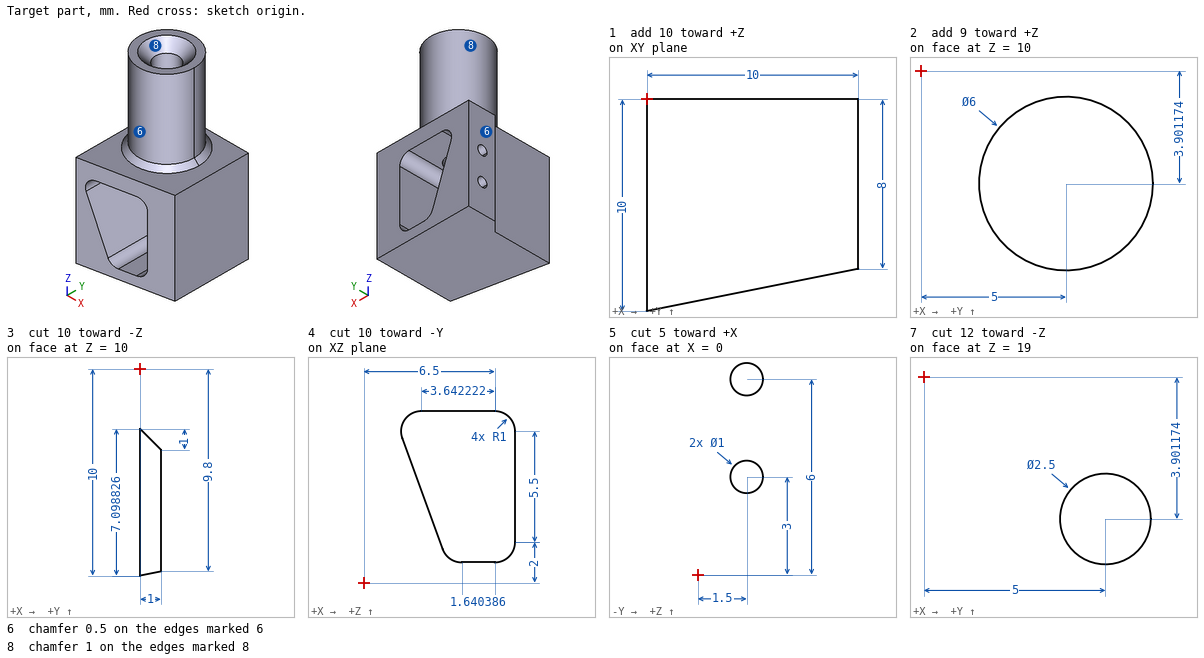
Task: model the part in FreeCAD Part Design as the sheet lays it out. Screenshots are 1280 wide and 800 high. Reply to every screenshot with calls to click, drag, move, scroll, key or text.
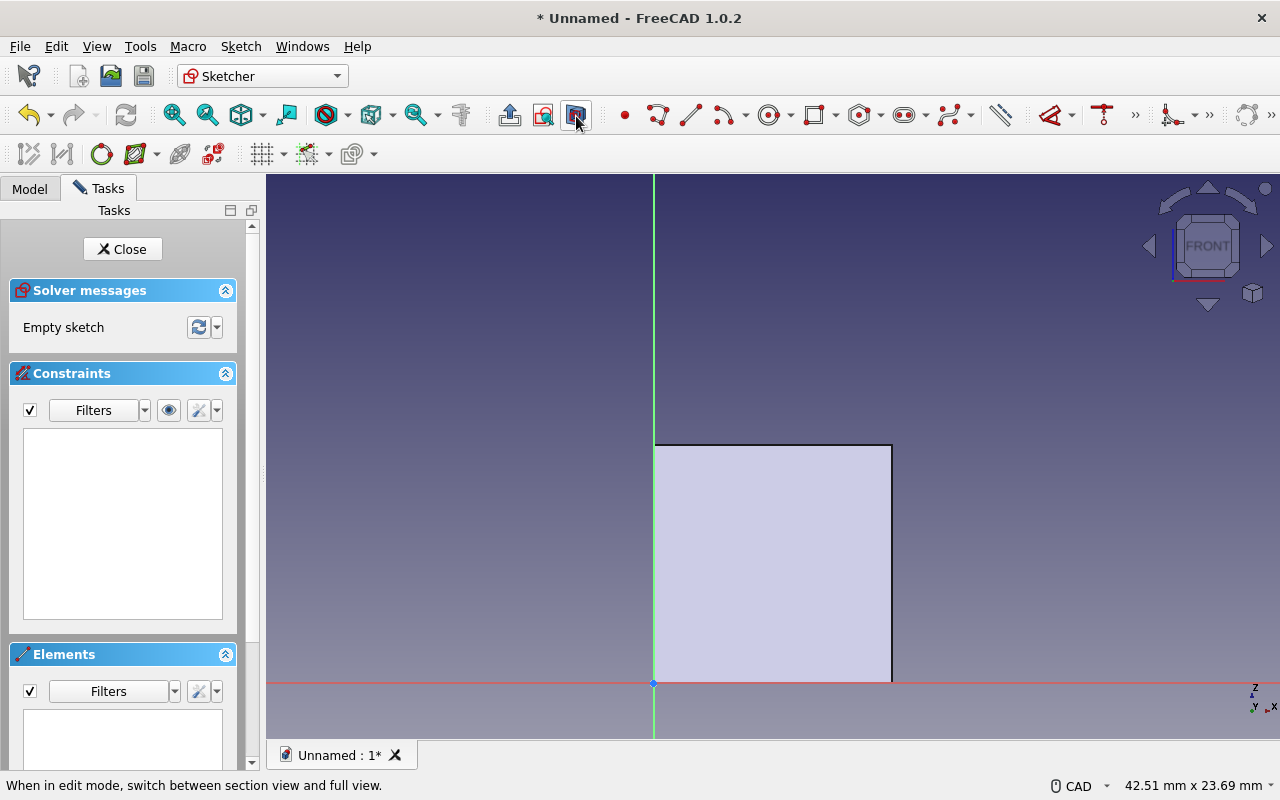
scroll(790, 711, up, 3)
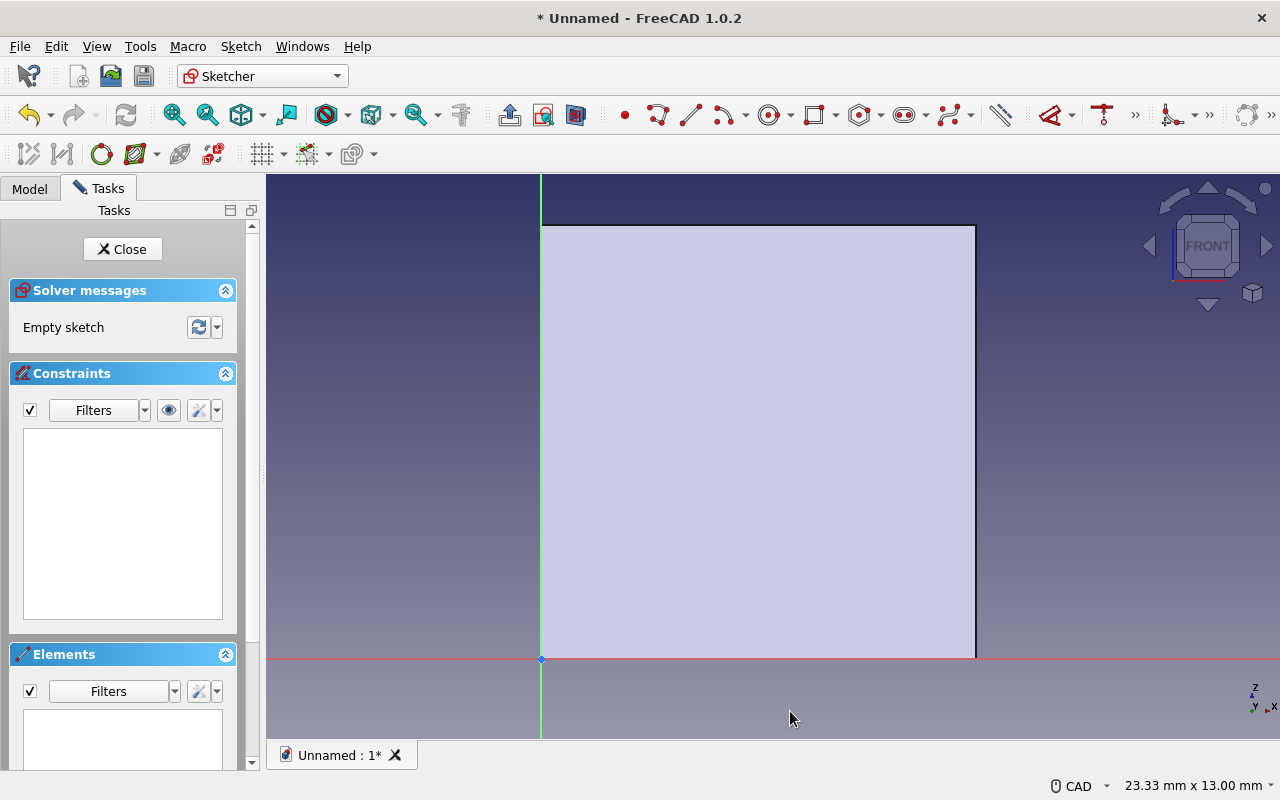
click(691, 116)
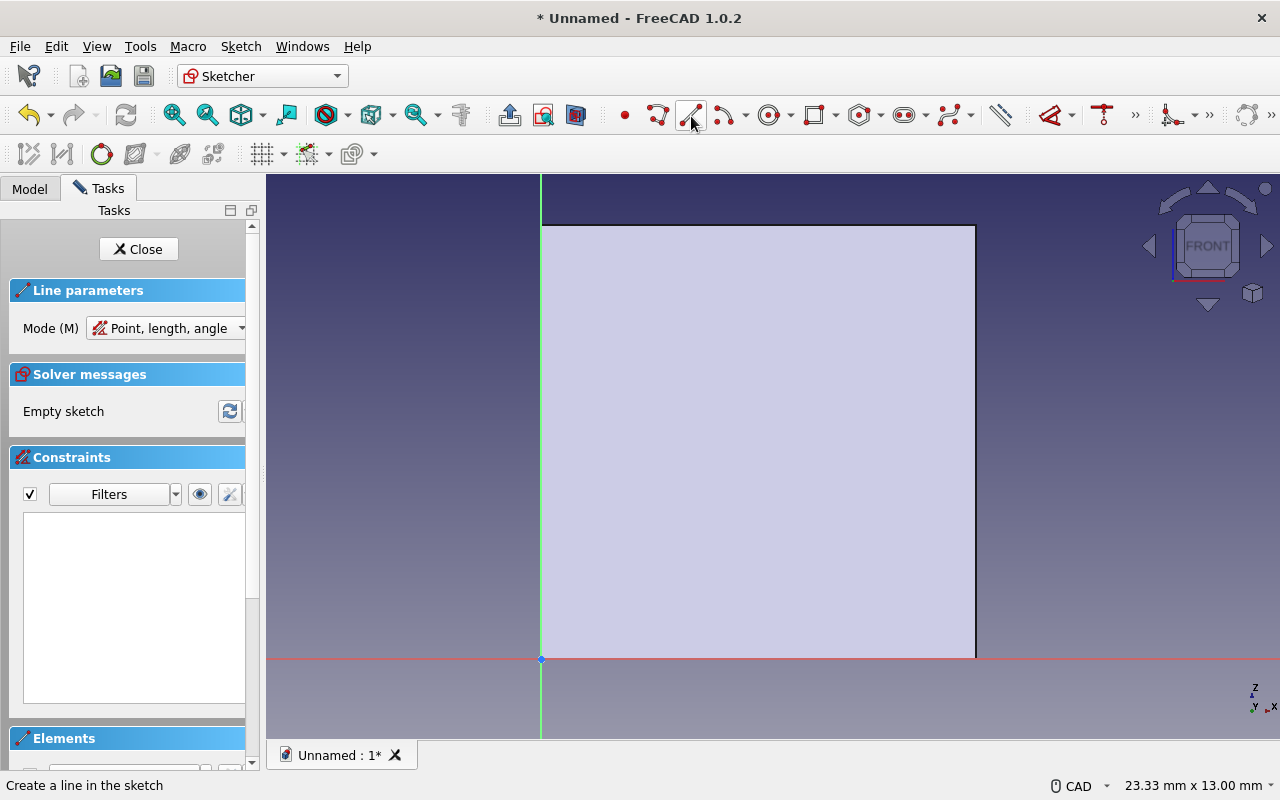
click(712, 587)
click(625, 348)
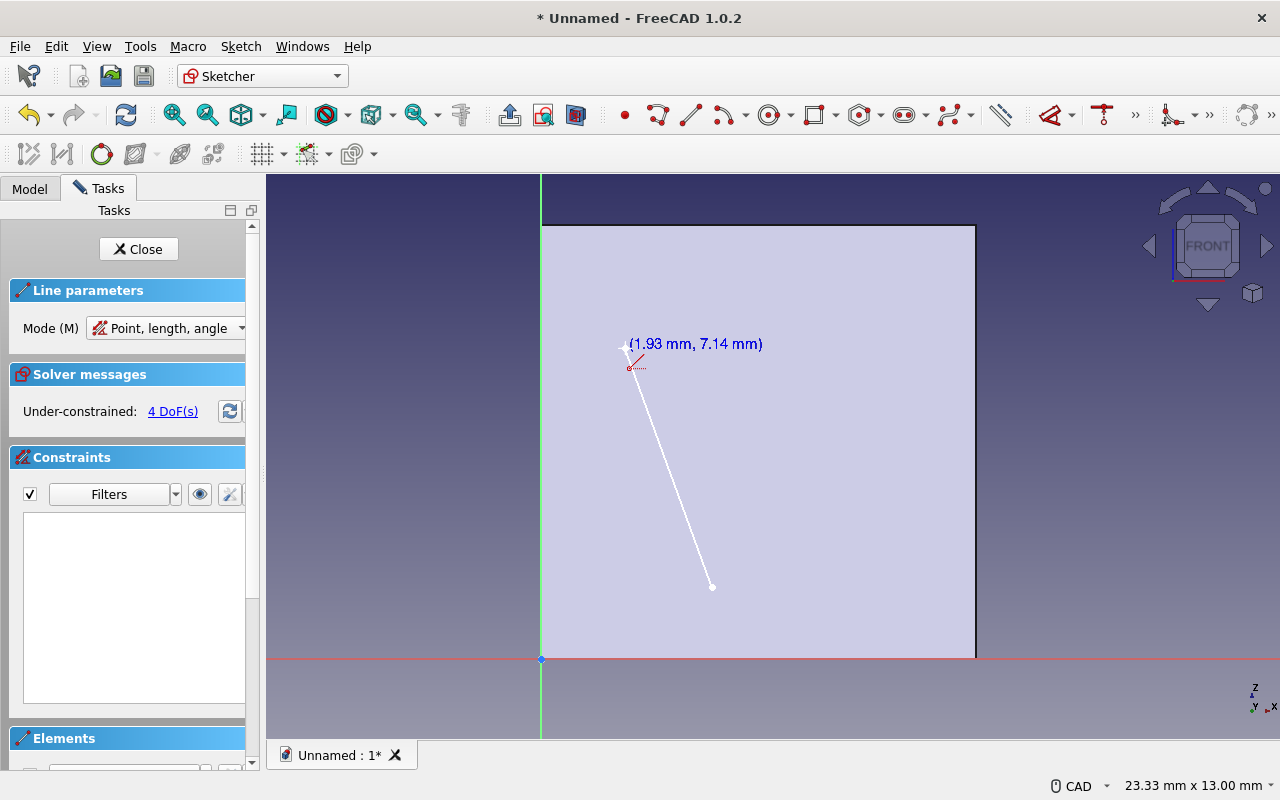
click(665, 290)
click(824, 290)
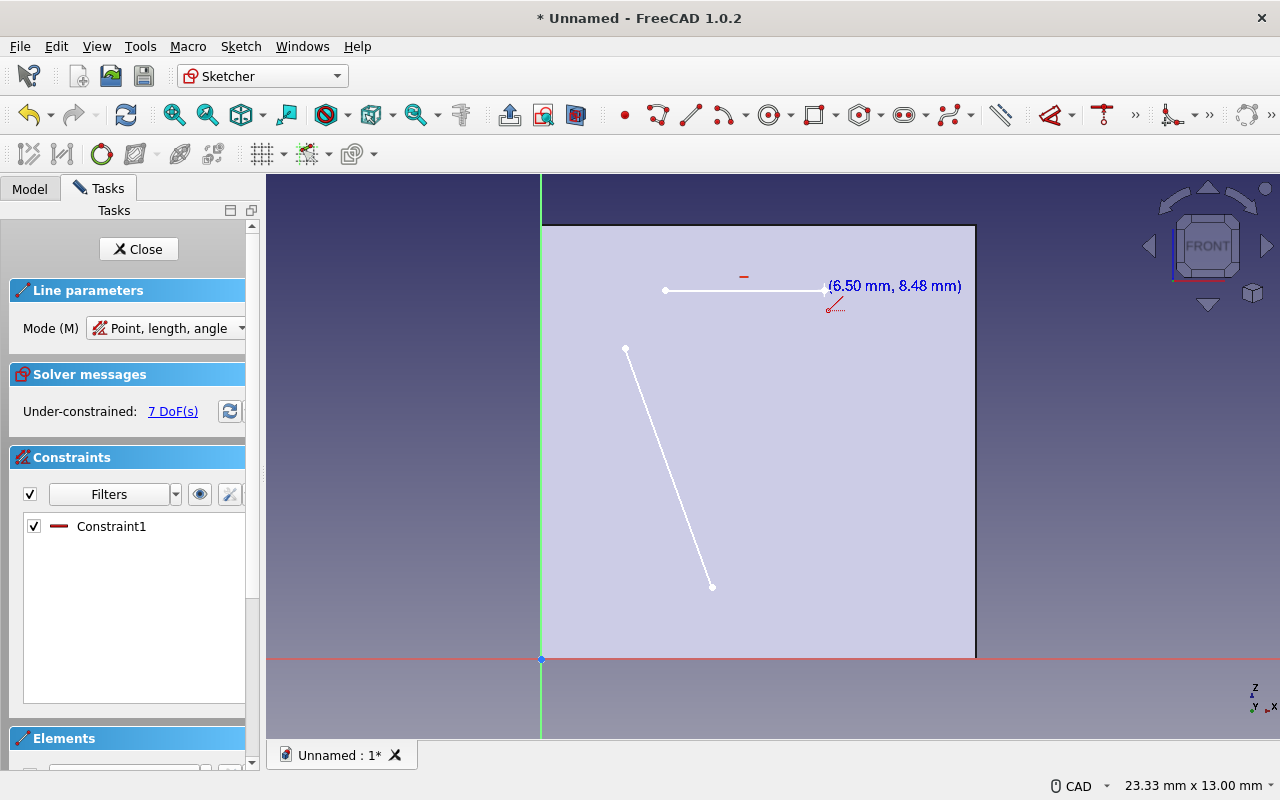
click(867, 333)
click(867, 572)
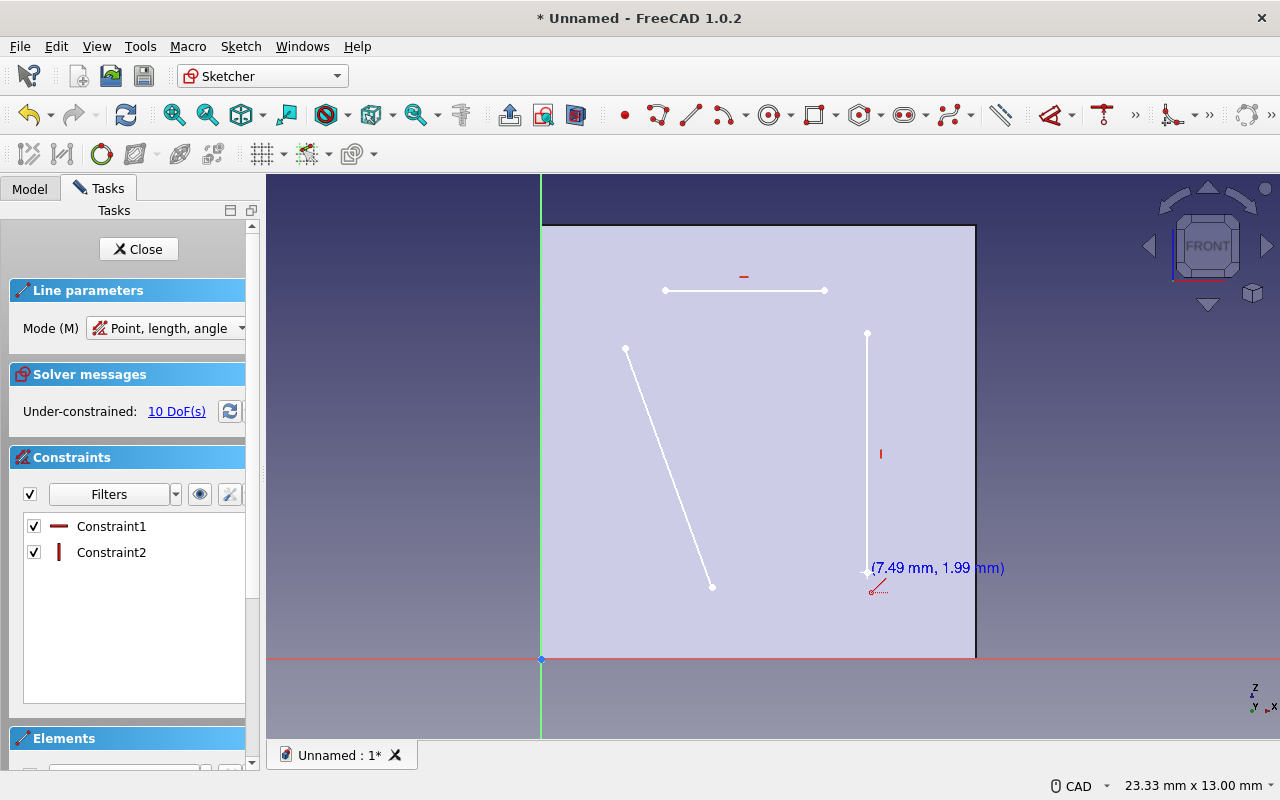
click(824, 616)
click(752, 616)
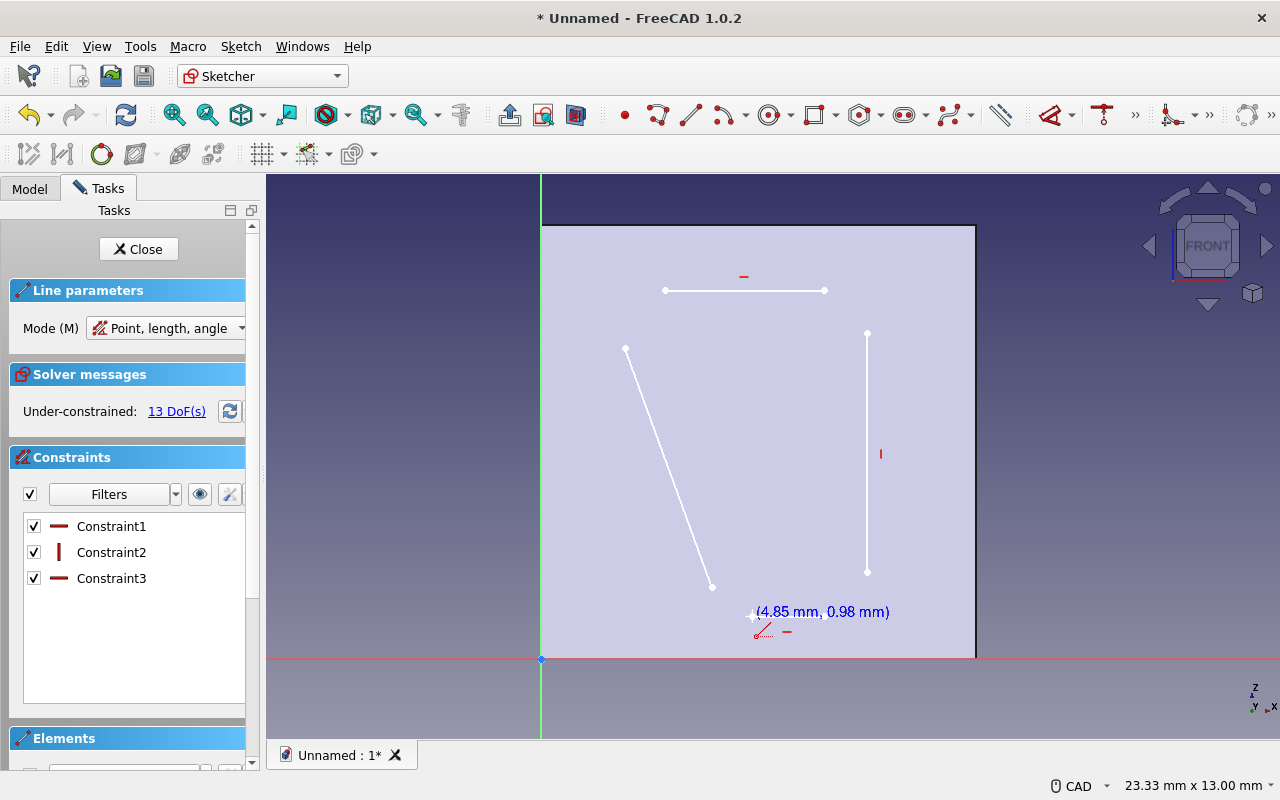
key(g)
key(3)
key(a)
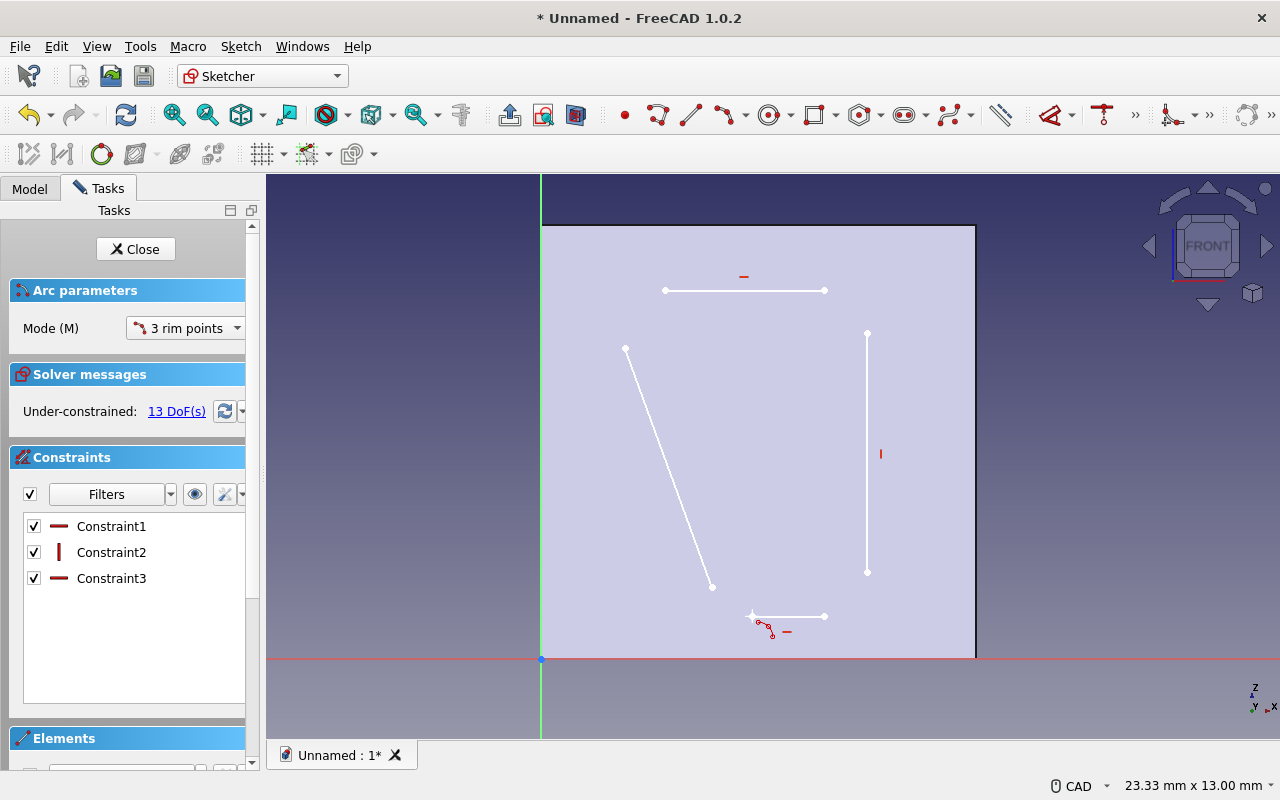
click(625, 349)
click(665, 291)
click(630, 308)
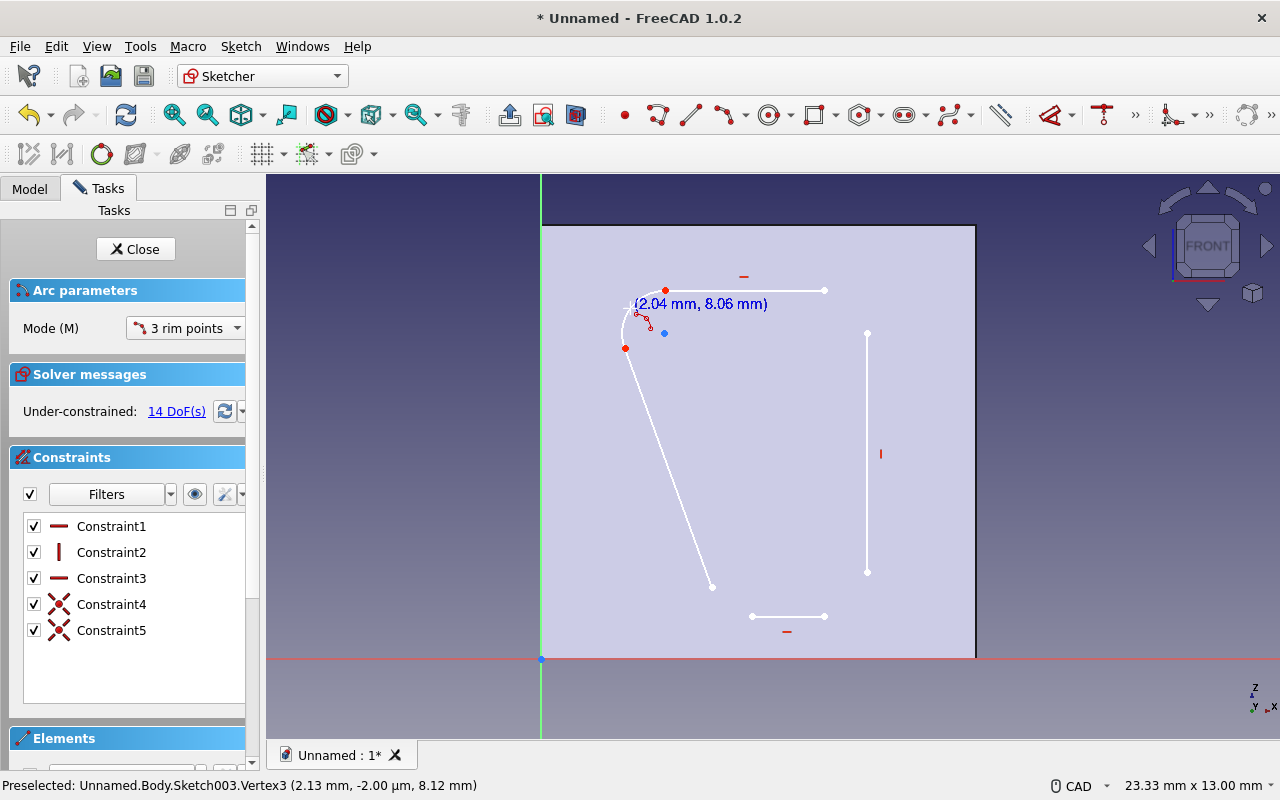
click(824, 291)
click(867, 334)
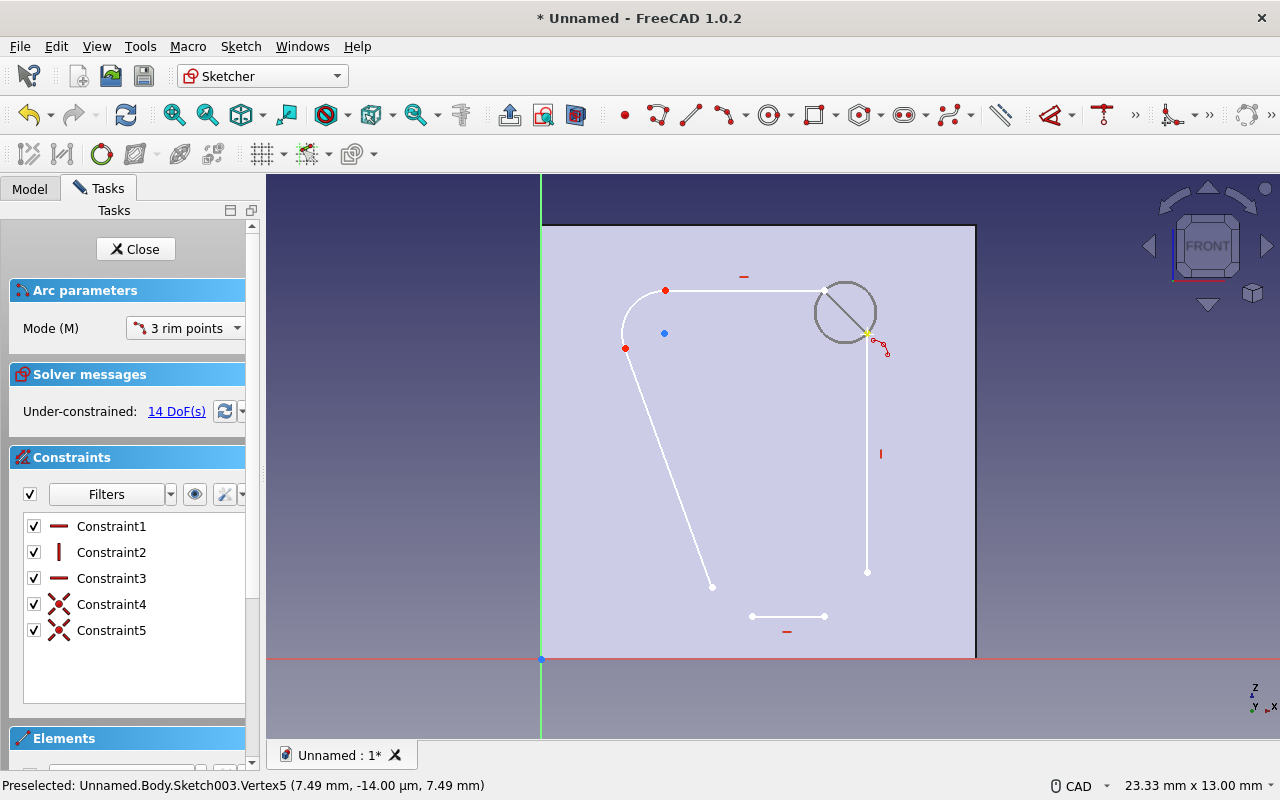
scroll(855, 303, up, 2)